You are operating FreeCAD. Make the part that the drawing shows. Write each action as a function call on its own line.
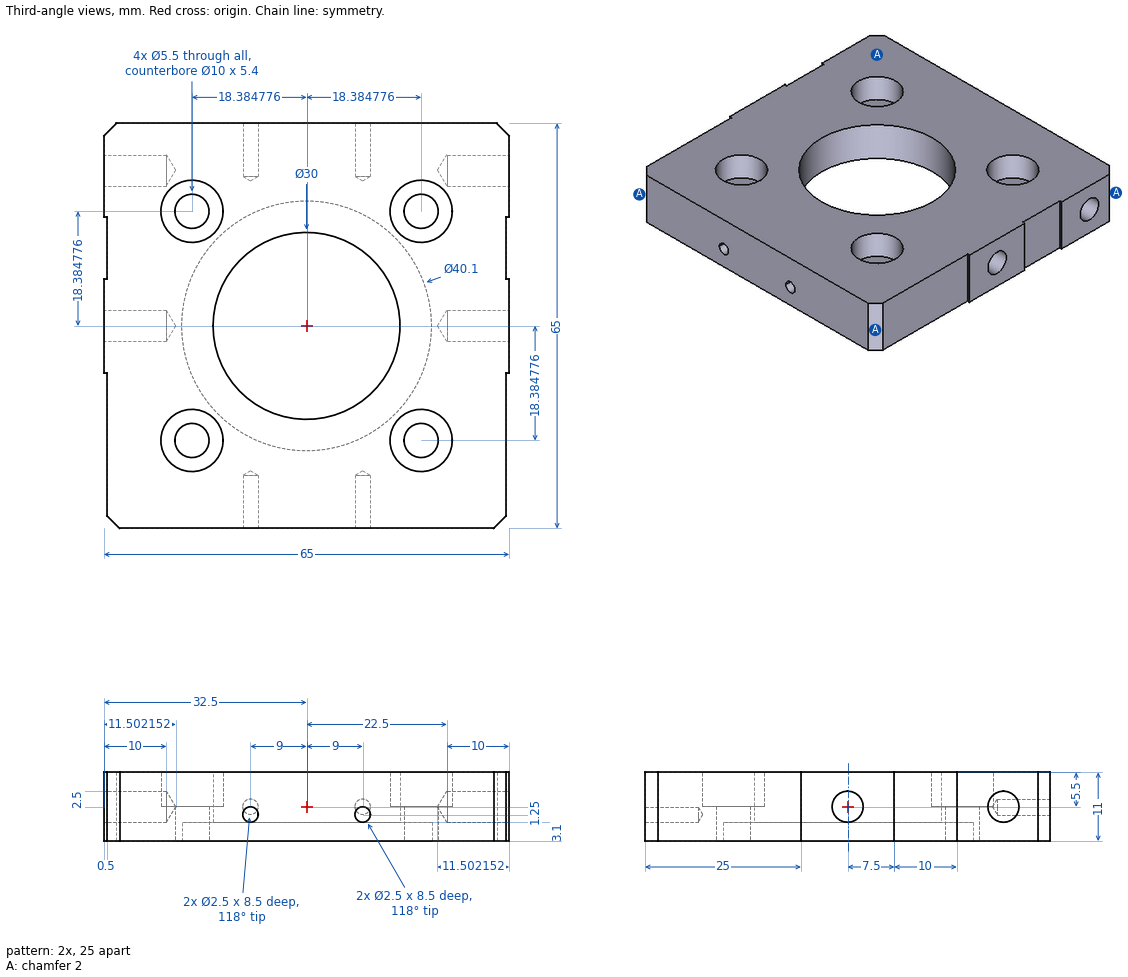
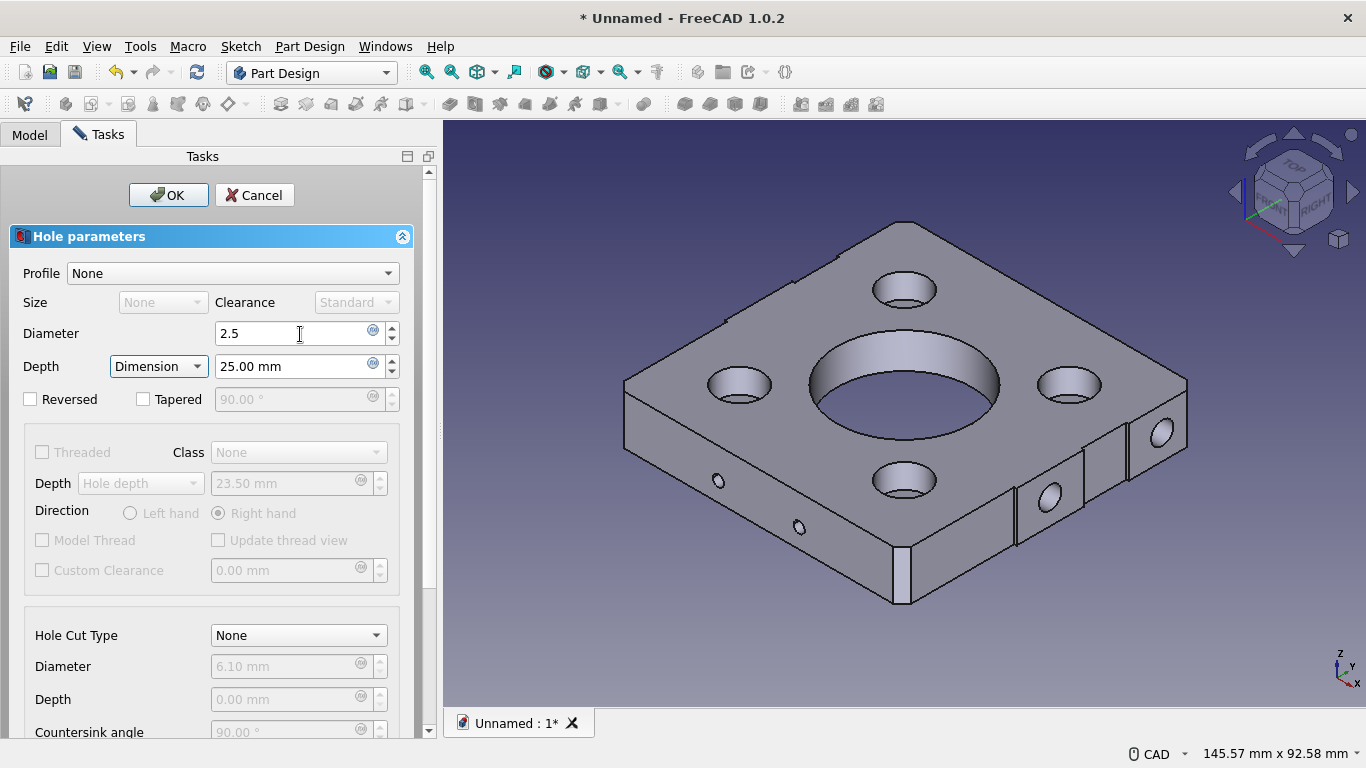
triple_click(300, 366)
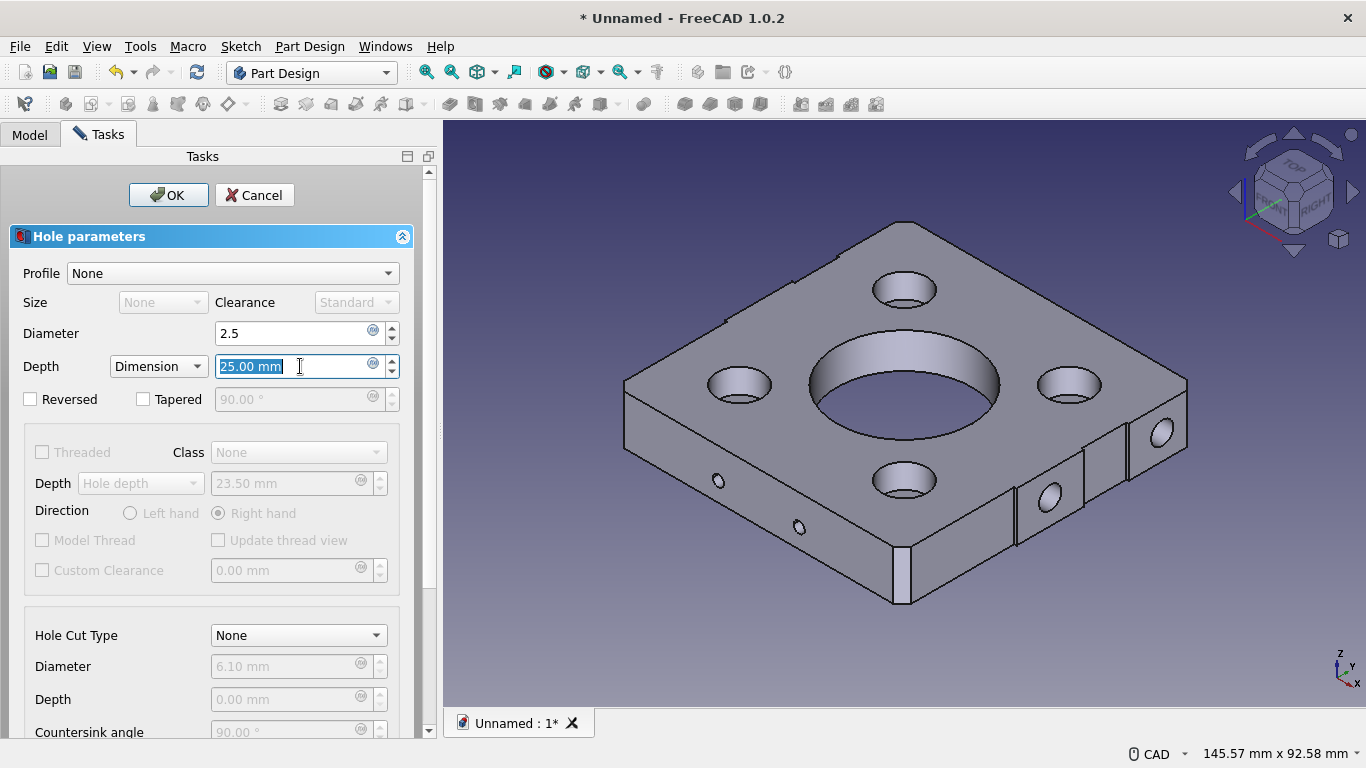
text(8.5)
key(Tab)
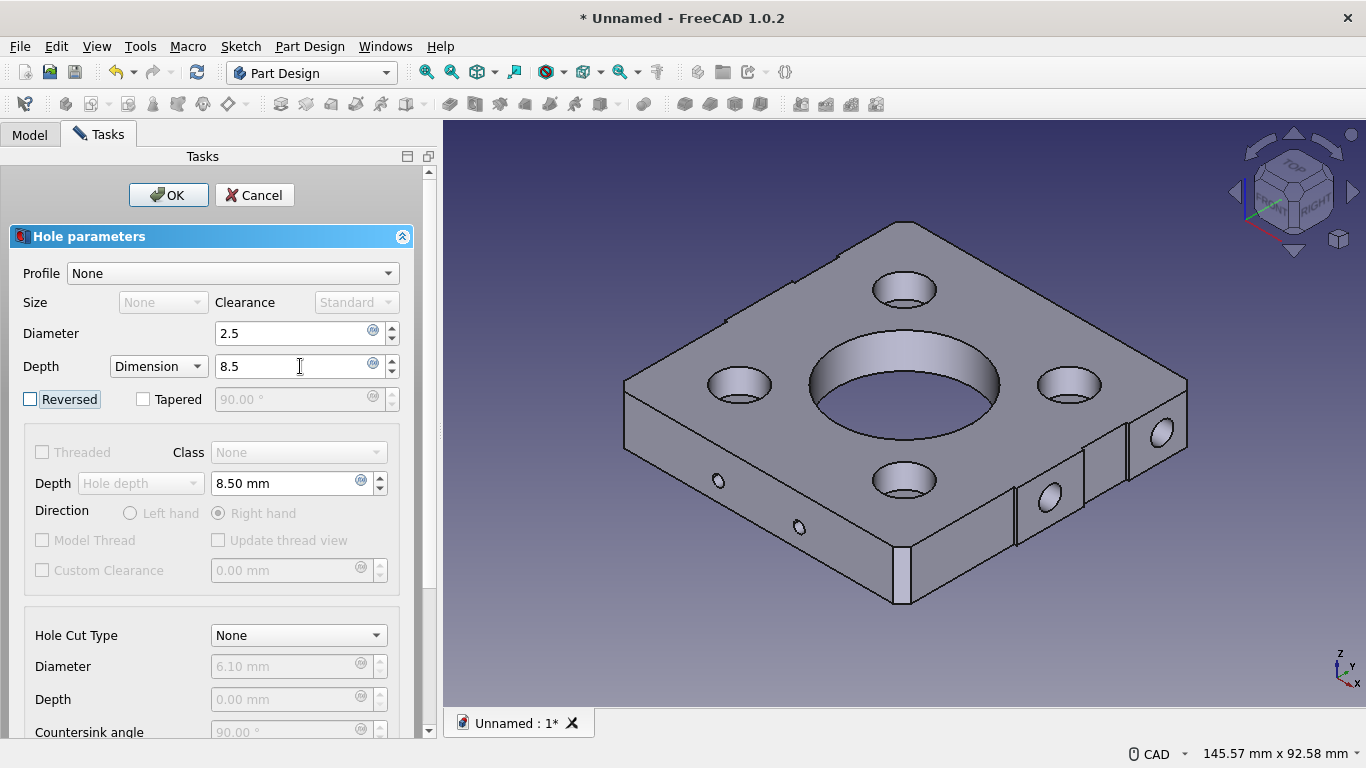
click(169, 195)